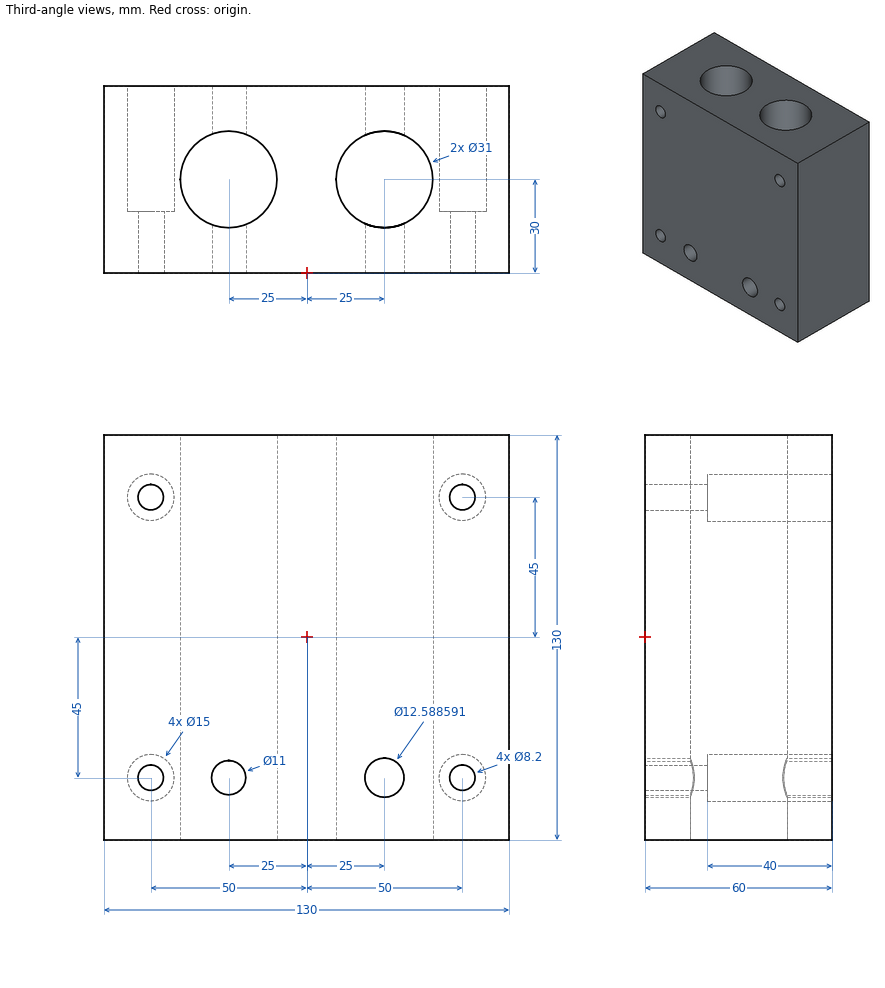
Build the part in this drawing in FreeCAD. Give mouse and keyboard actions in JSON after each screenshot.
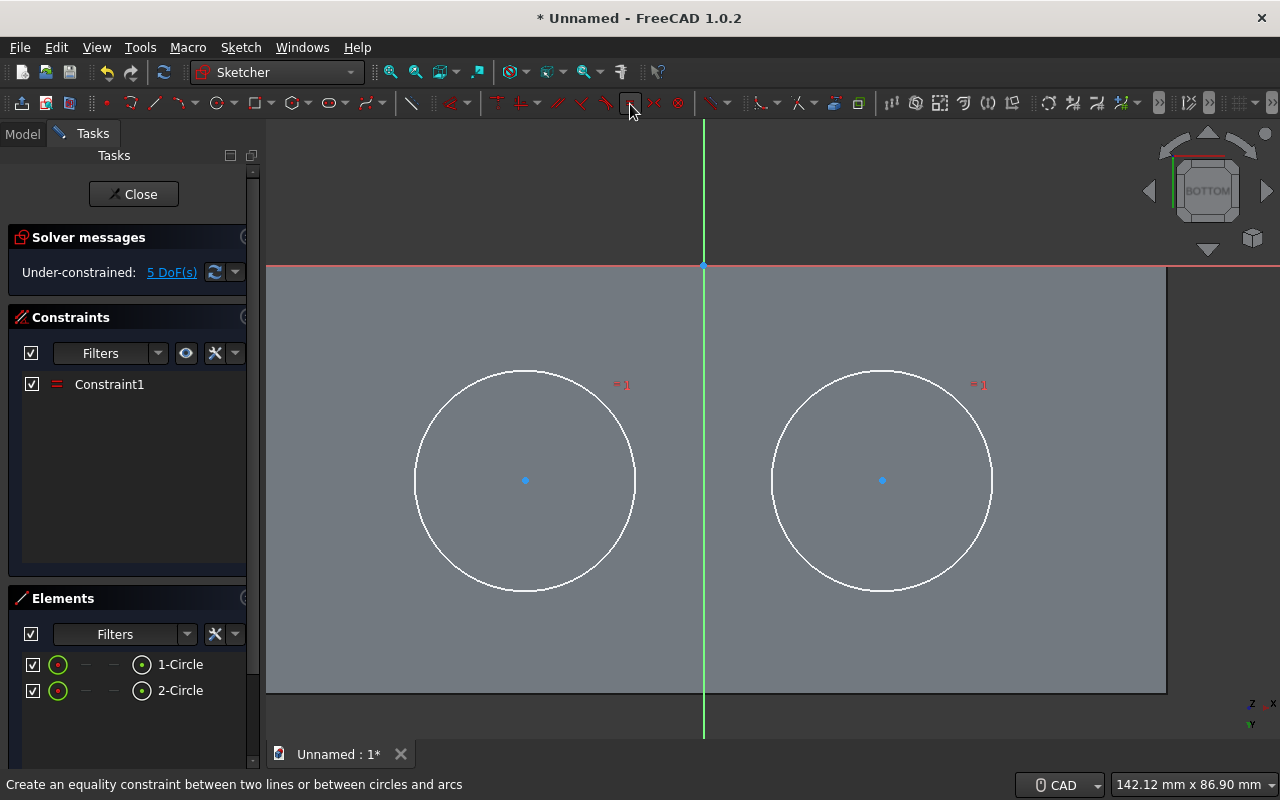
{"action": "left_click", "coordinate": [882, 481]}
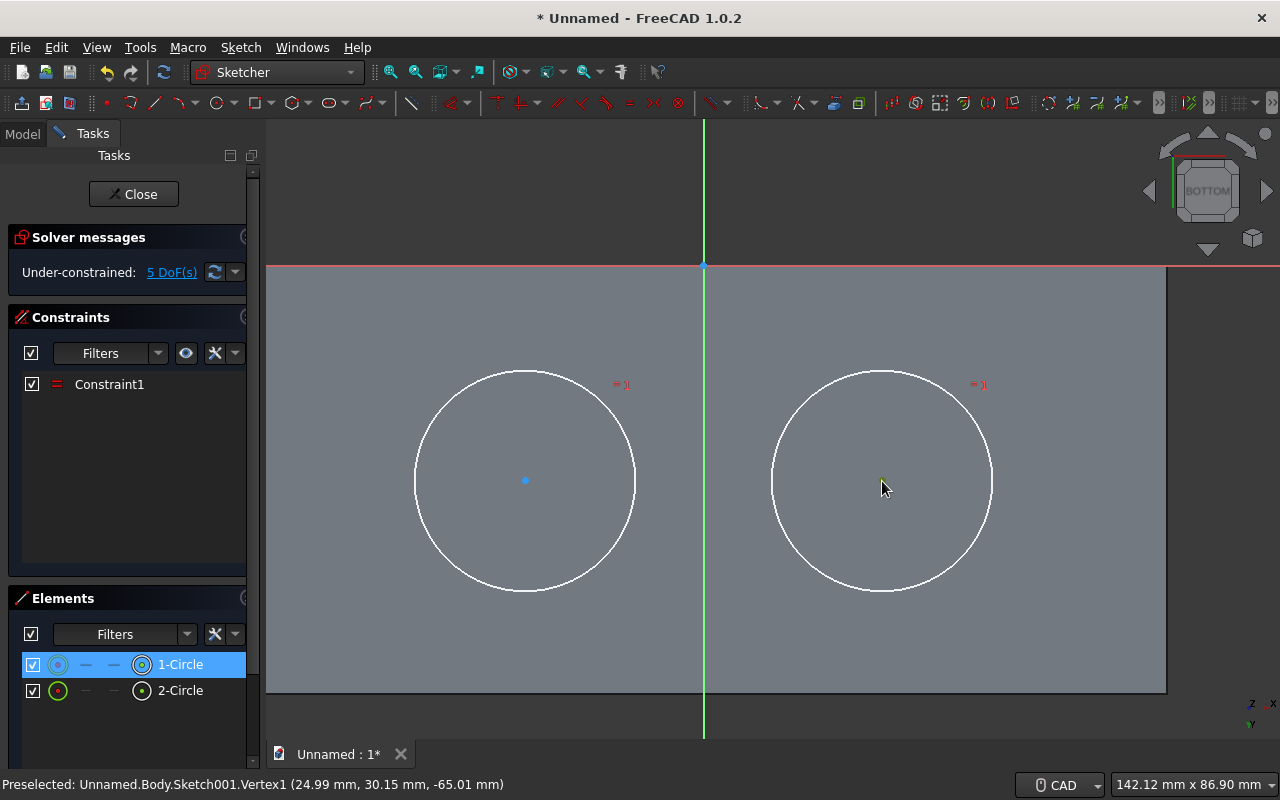
{"action": "left_click", "coordinate": [525, 481]}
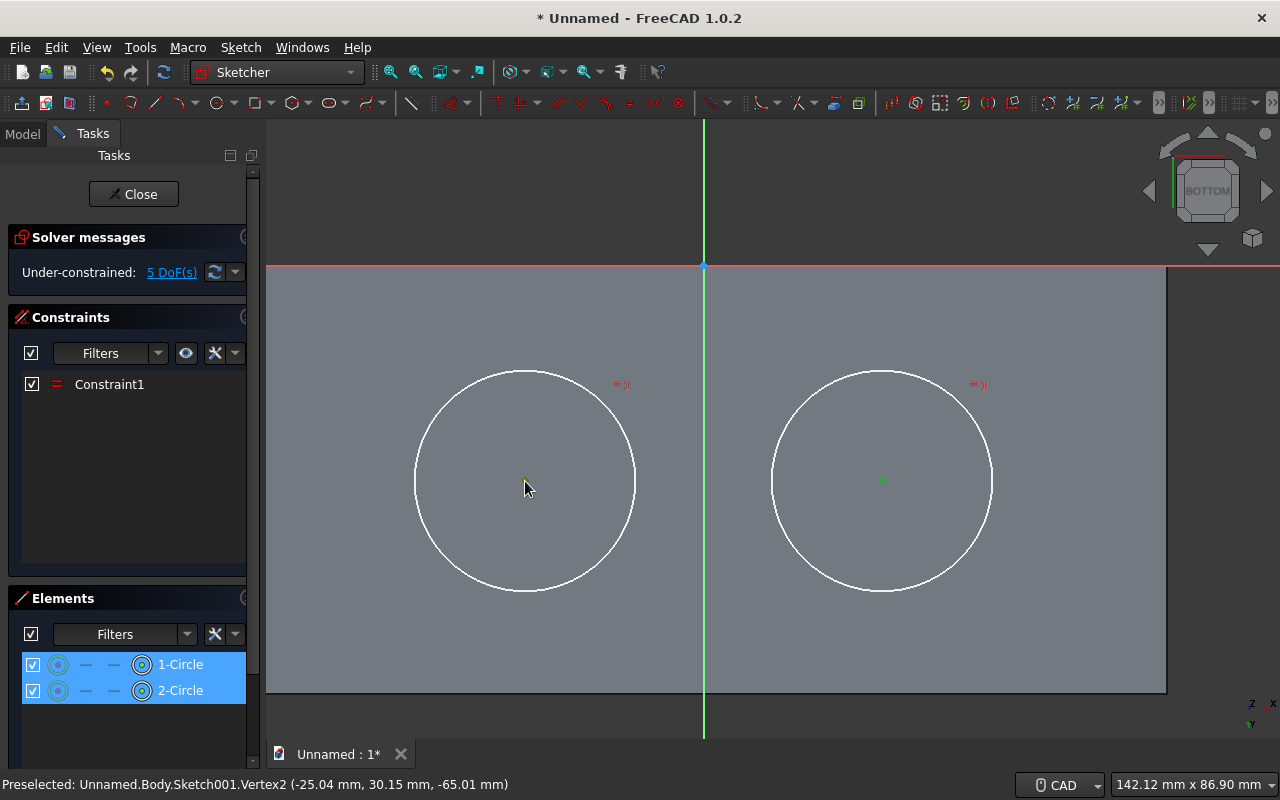
{"action": "key", "text": "h"}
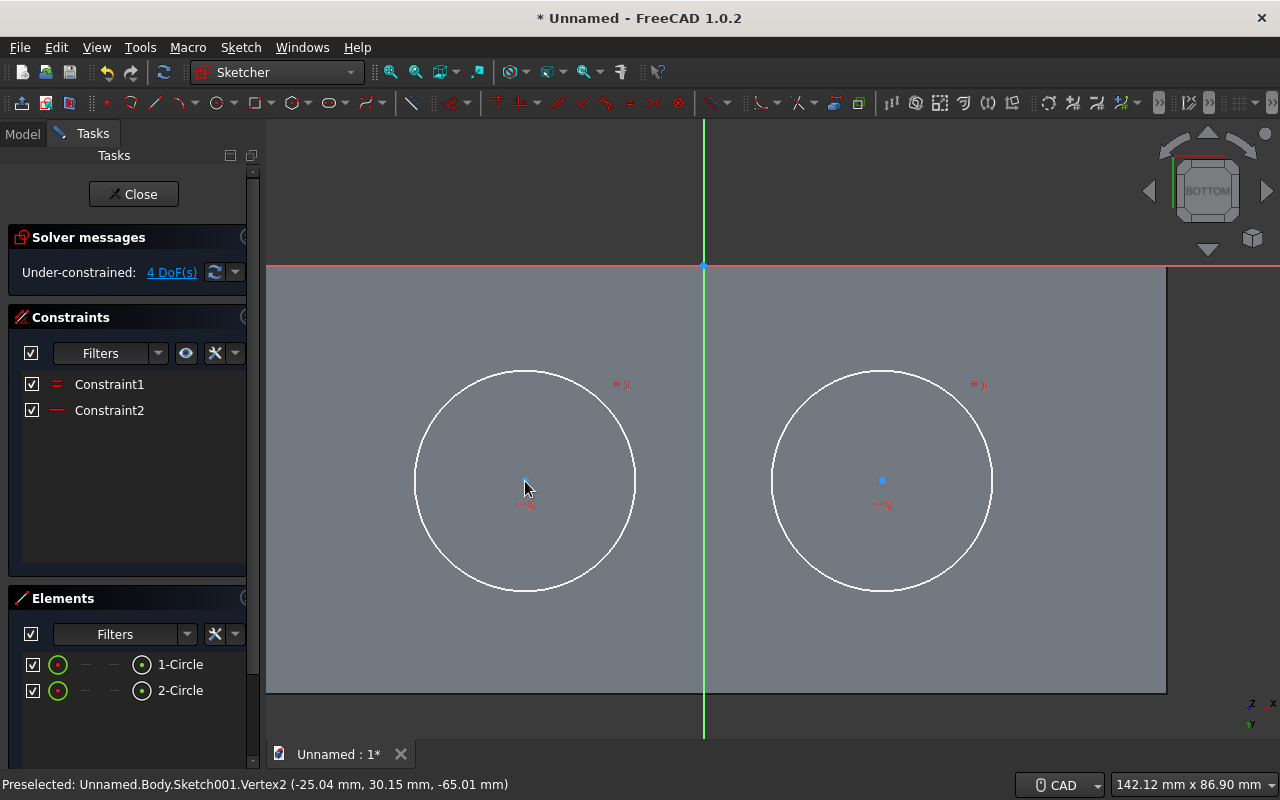
{"action": "left_click", "coordinate": [960, 403]}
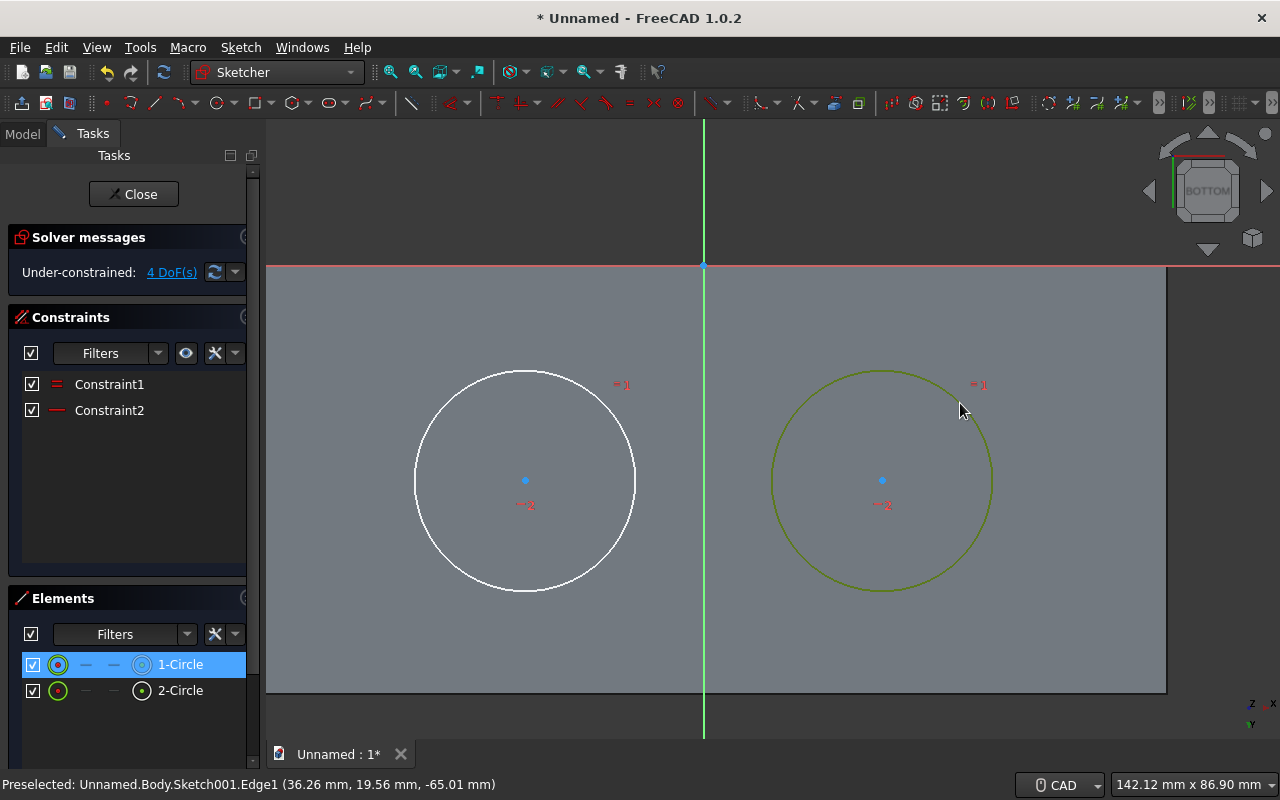
{"action": "key", "text": "k o"}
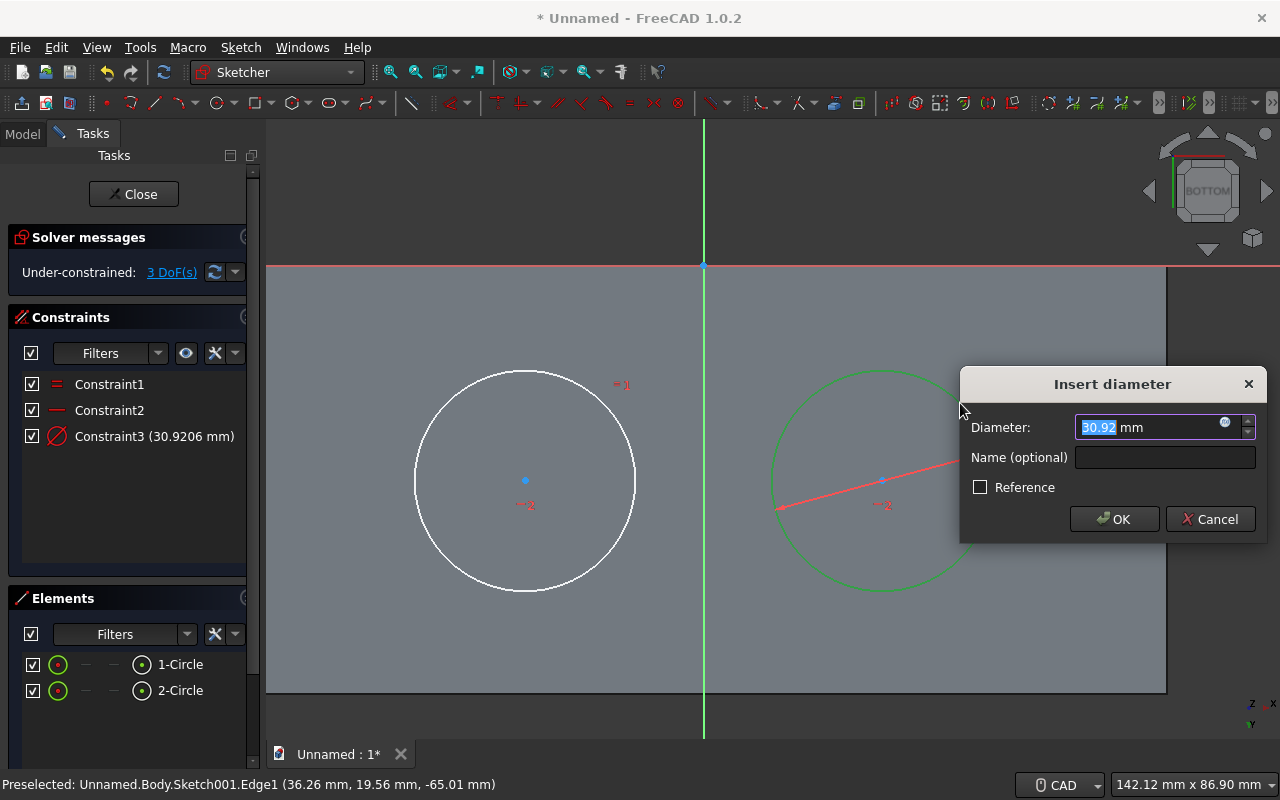
{"action": "type", "text": "31"}
{"action": "key", "text": "Return"}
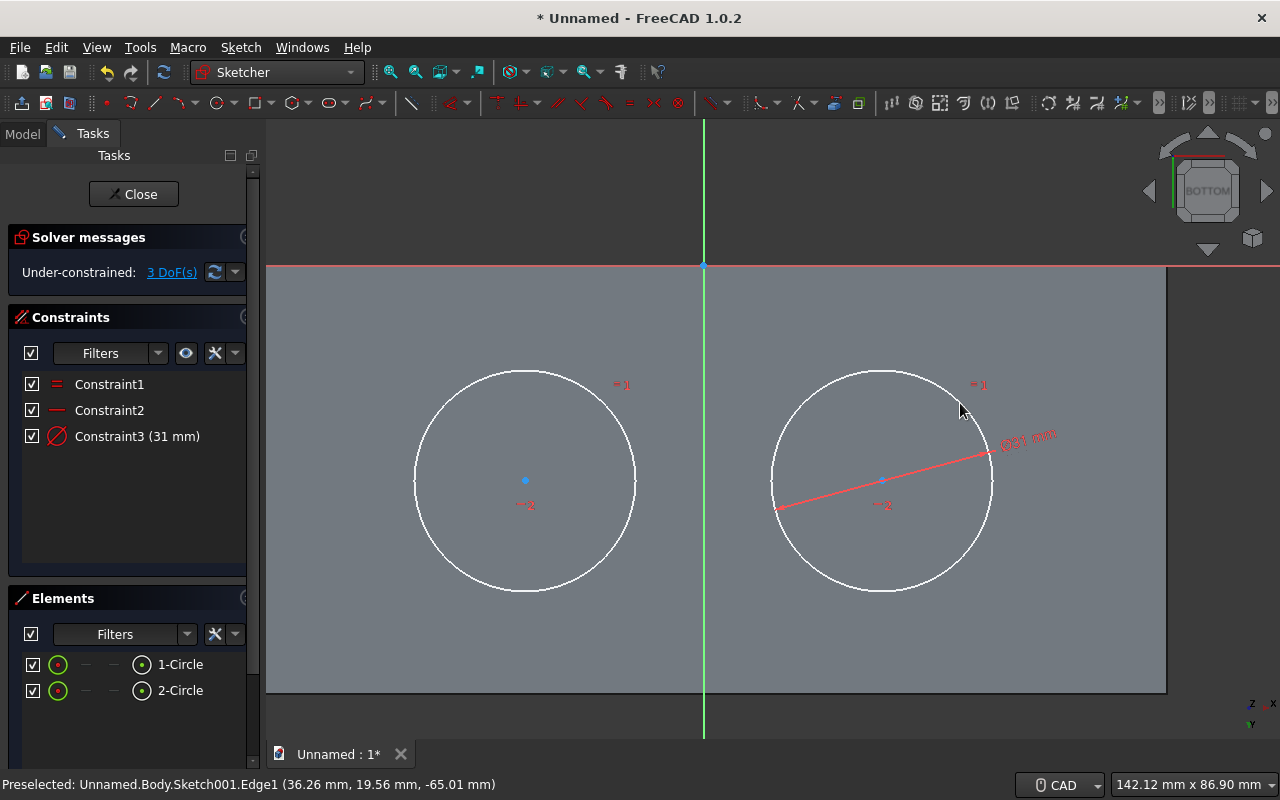
{"action": "left_click", "coordinate": [882, 481]}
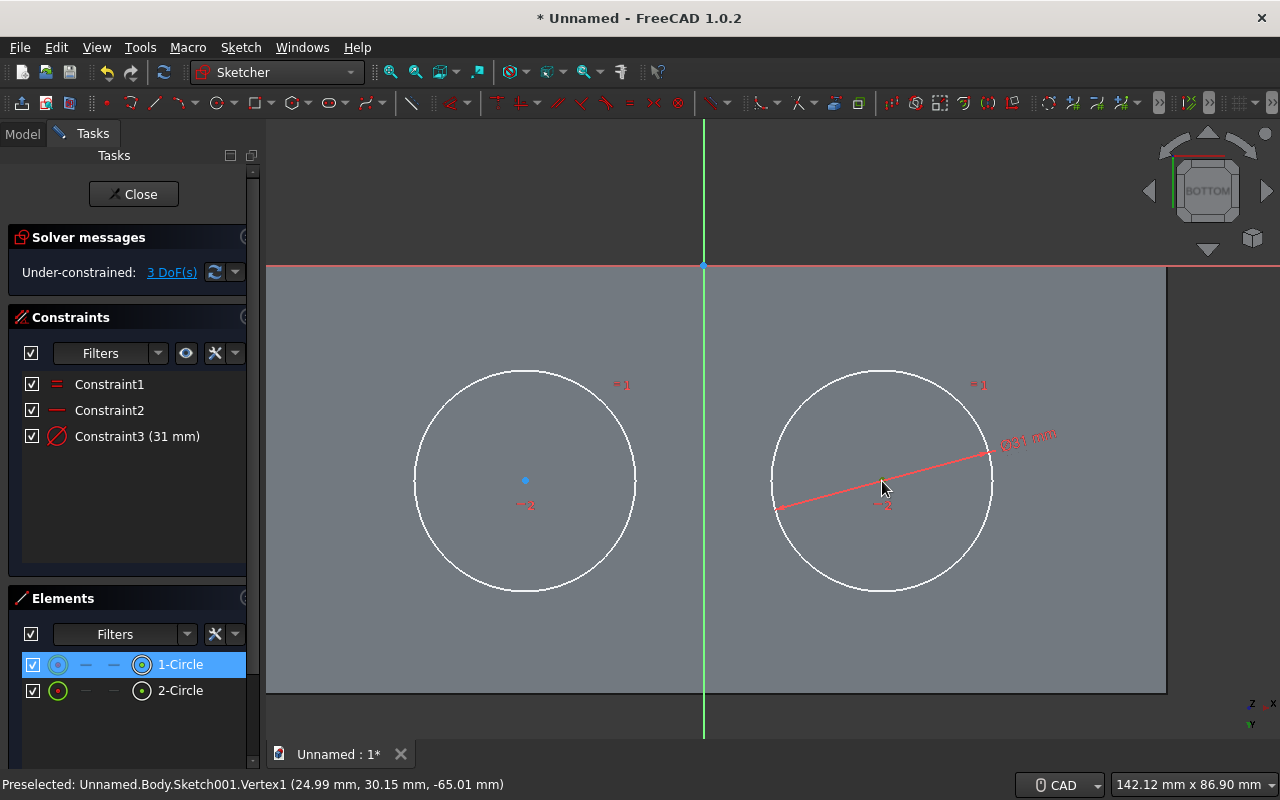
{"action": "key", "text": "l"}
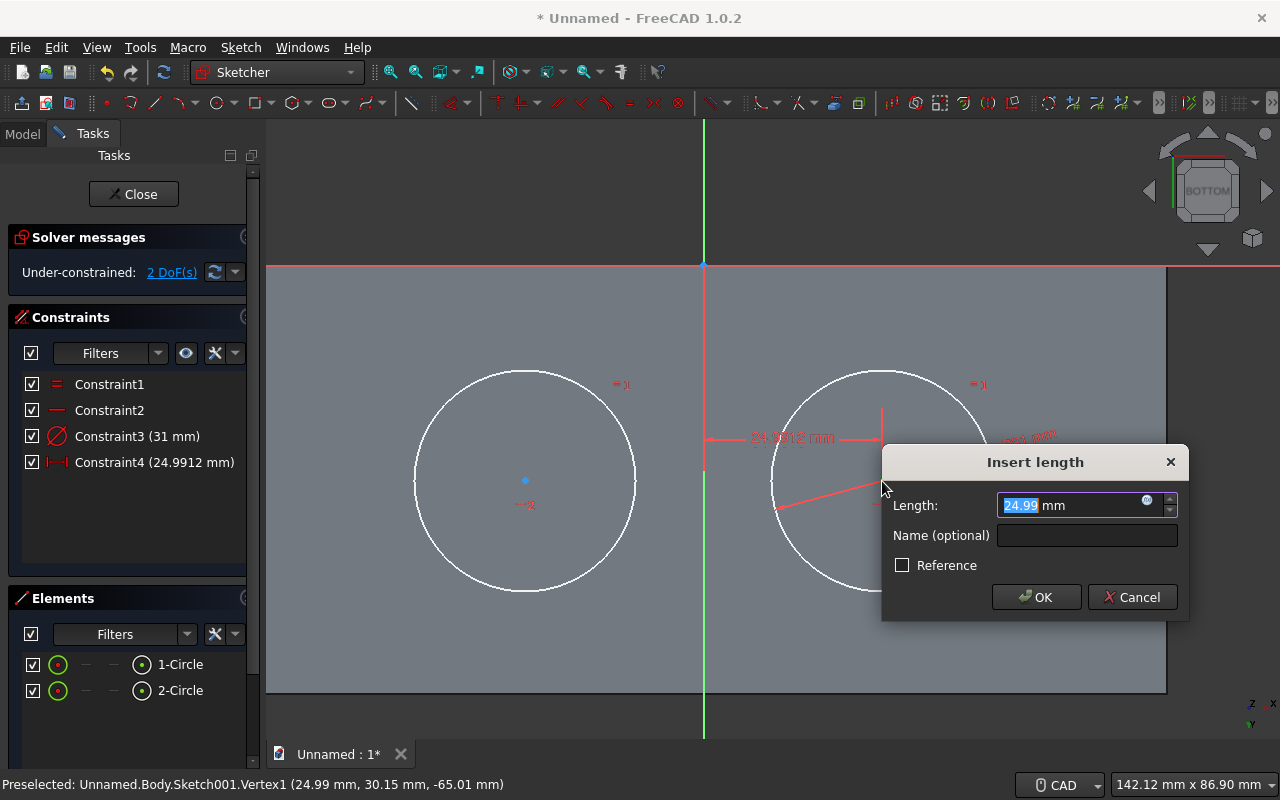
{"action": "type", "text": "25"}
{"action": "key", "text": "Return"}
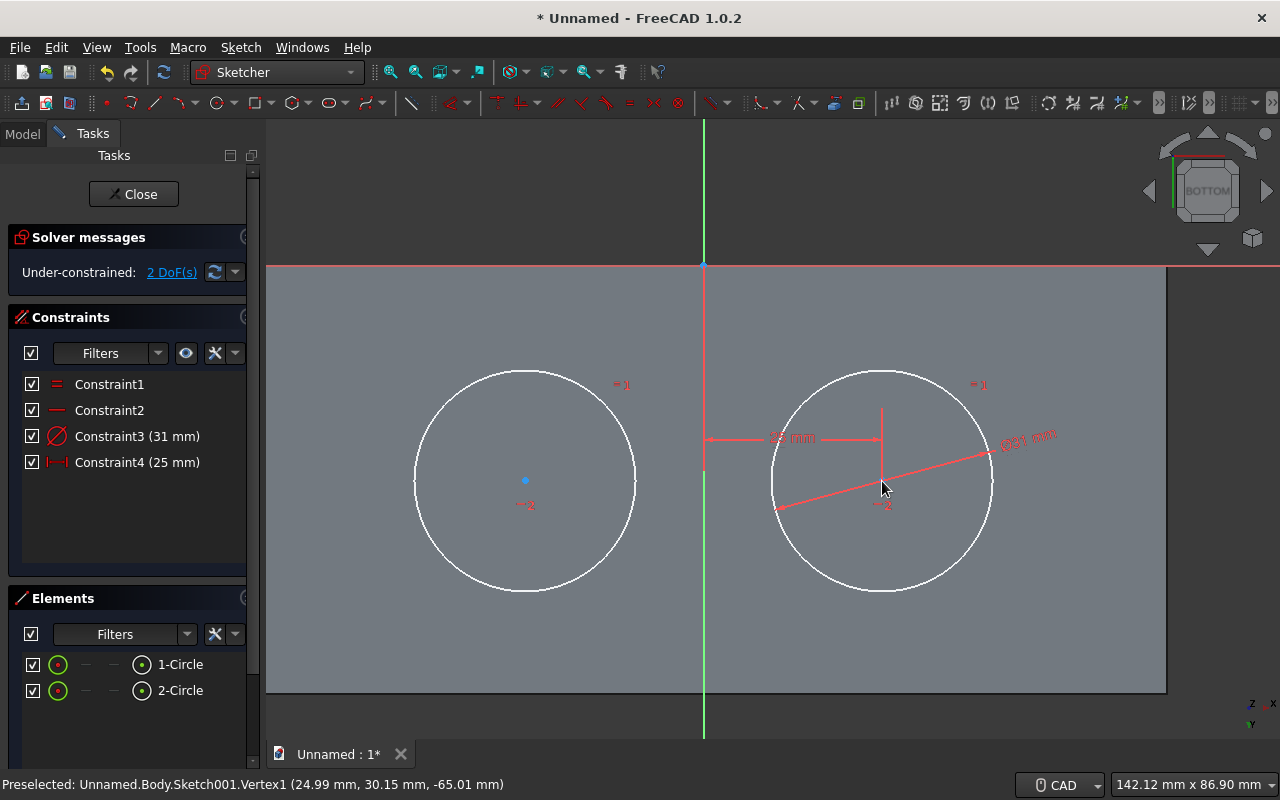
{"action": "left_click", "coordinate": [882, 481]}